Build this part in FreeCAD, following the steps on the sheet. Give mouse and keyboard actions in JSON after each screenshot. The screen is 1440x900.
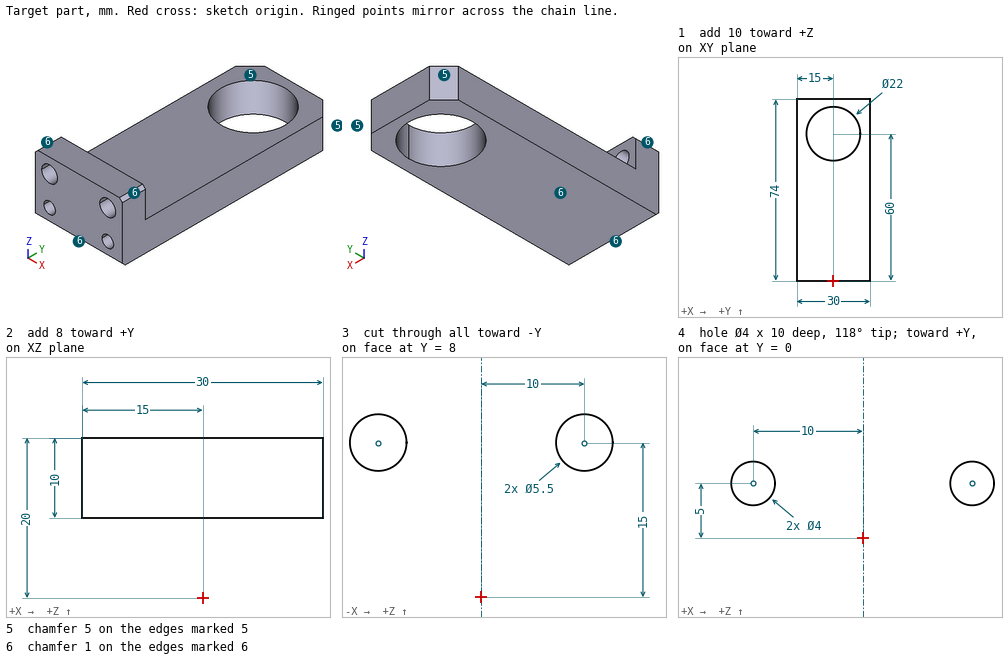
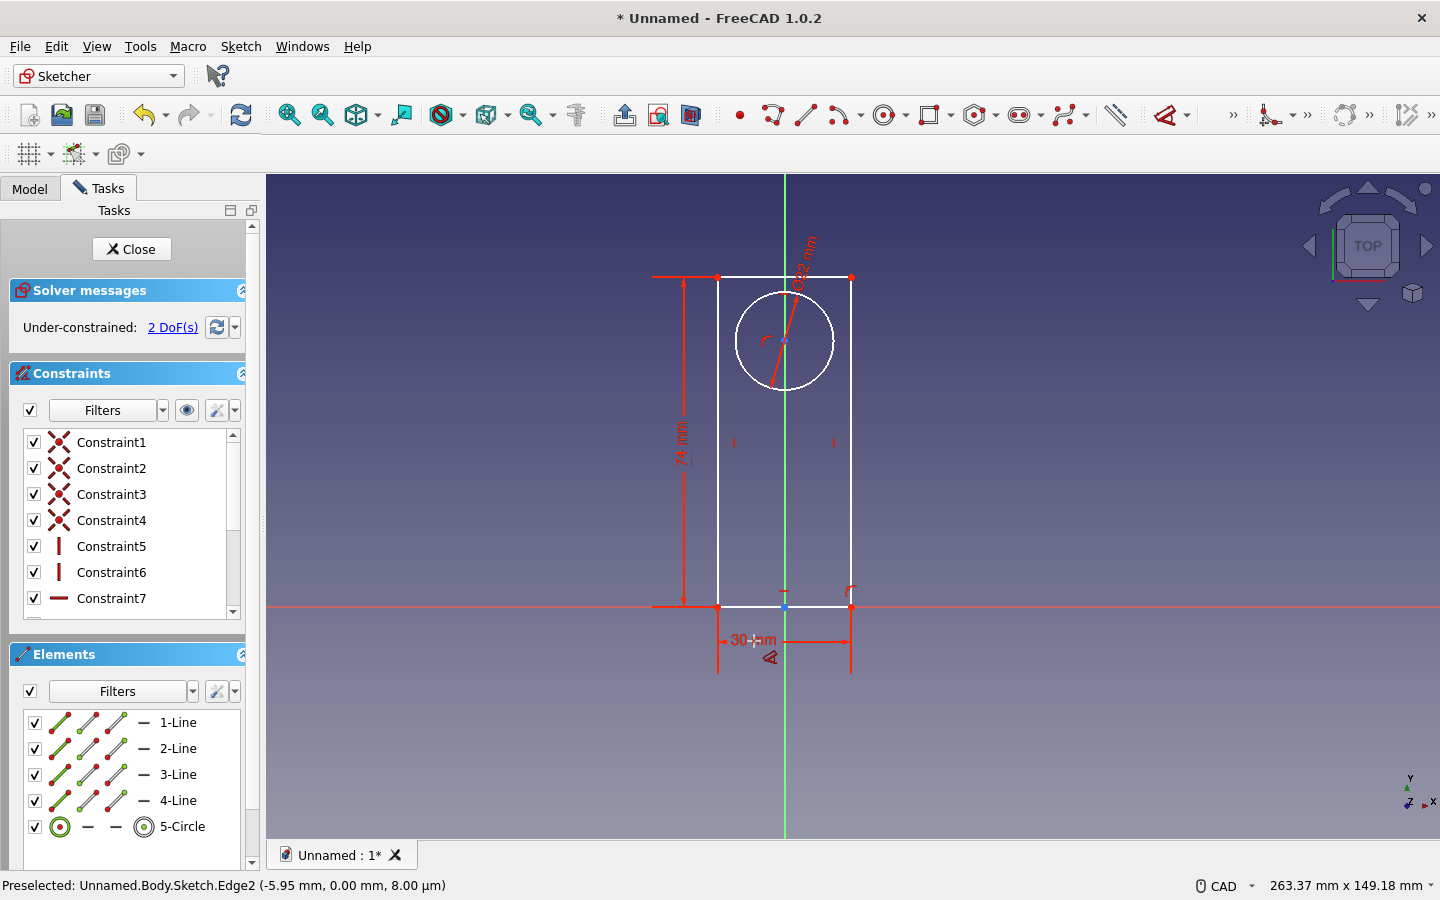
{"action": "left_click", "coordinate": [785, 341]}
{"action": "left_click", "coordinate": [819, 474]}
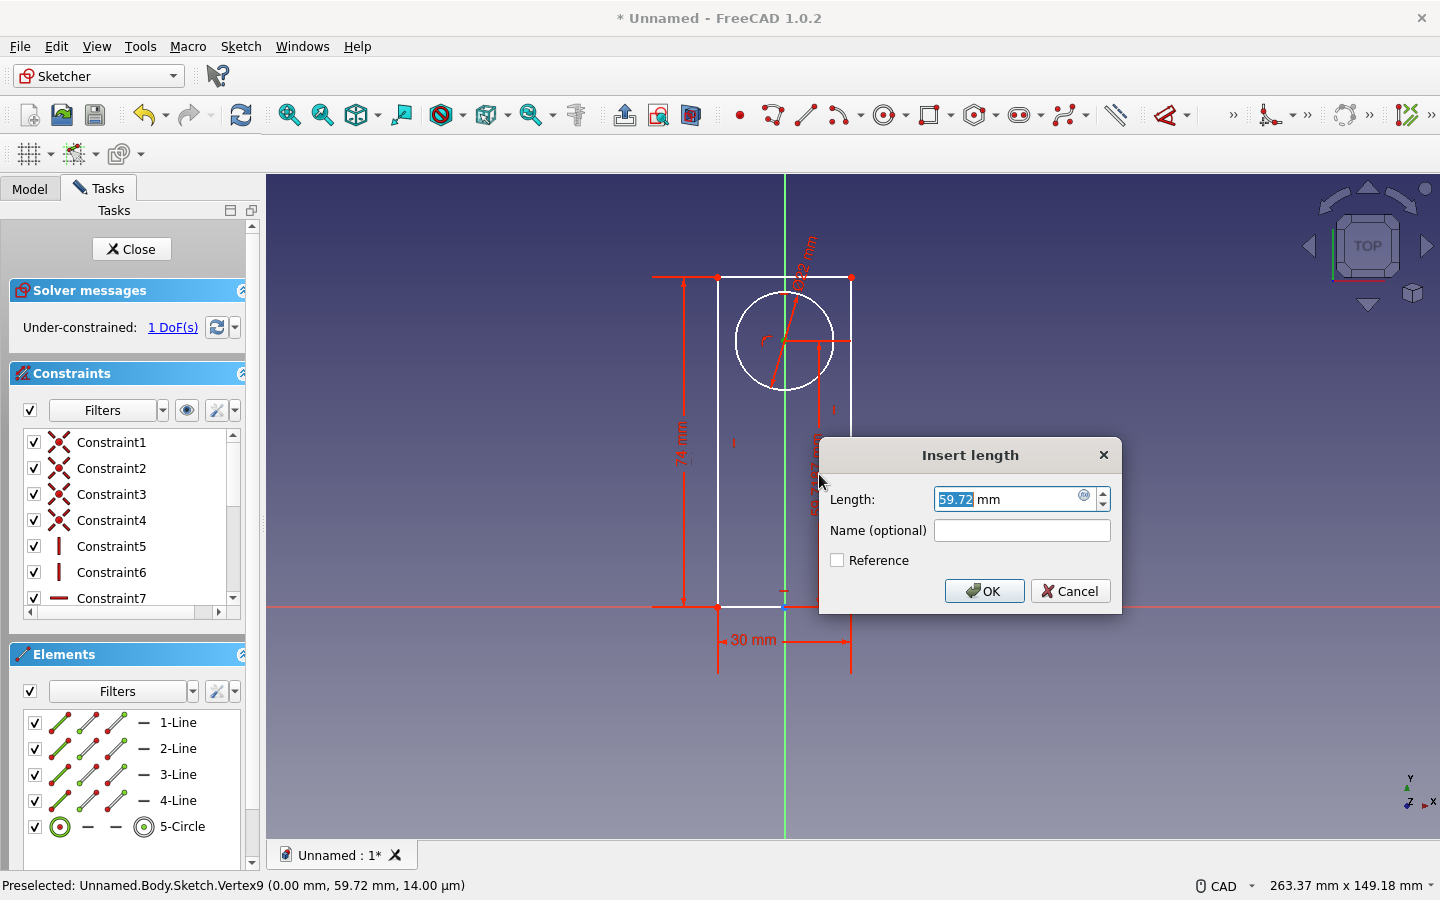
{"action": "type", "text": "60"}
{"action": "key", "text": "Return"}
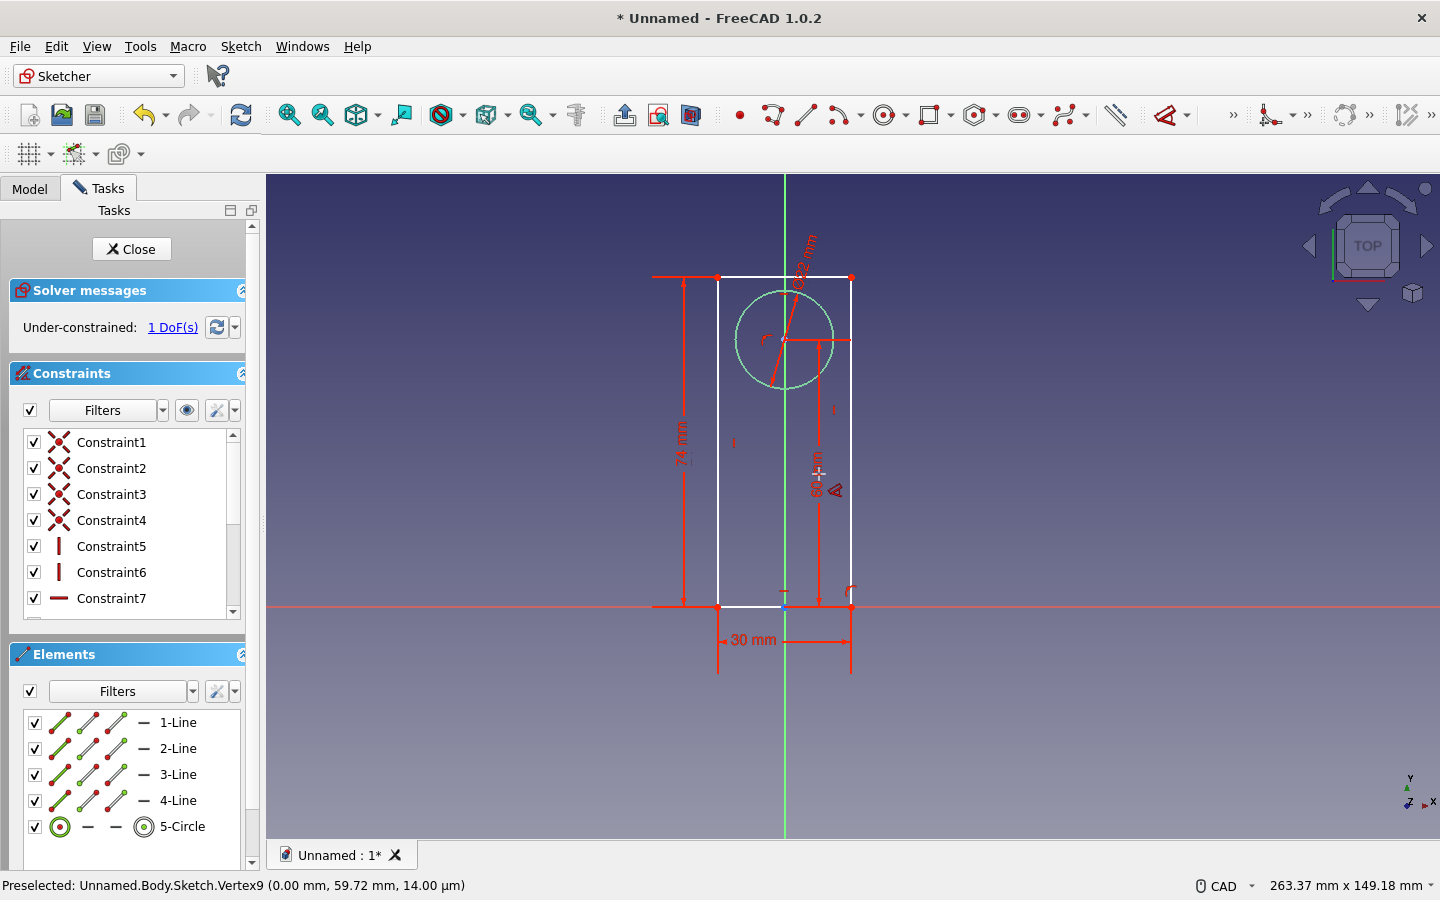
{"action": "left_click", "coordinate": [718, 277]}
{"action": "left_click", "coordinate": [736, 243]}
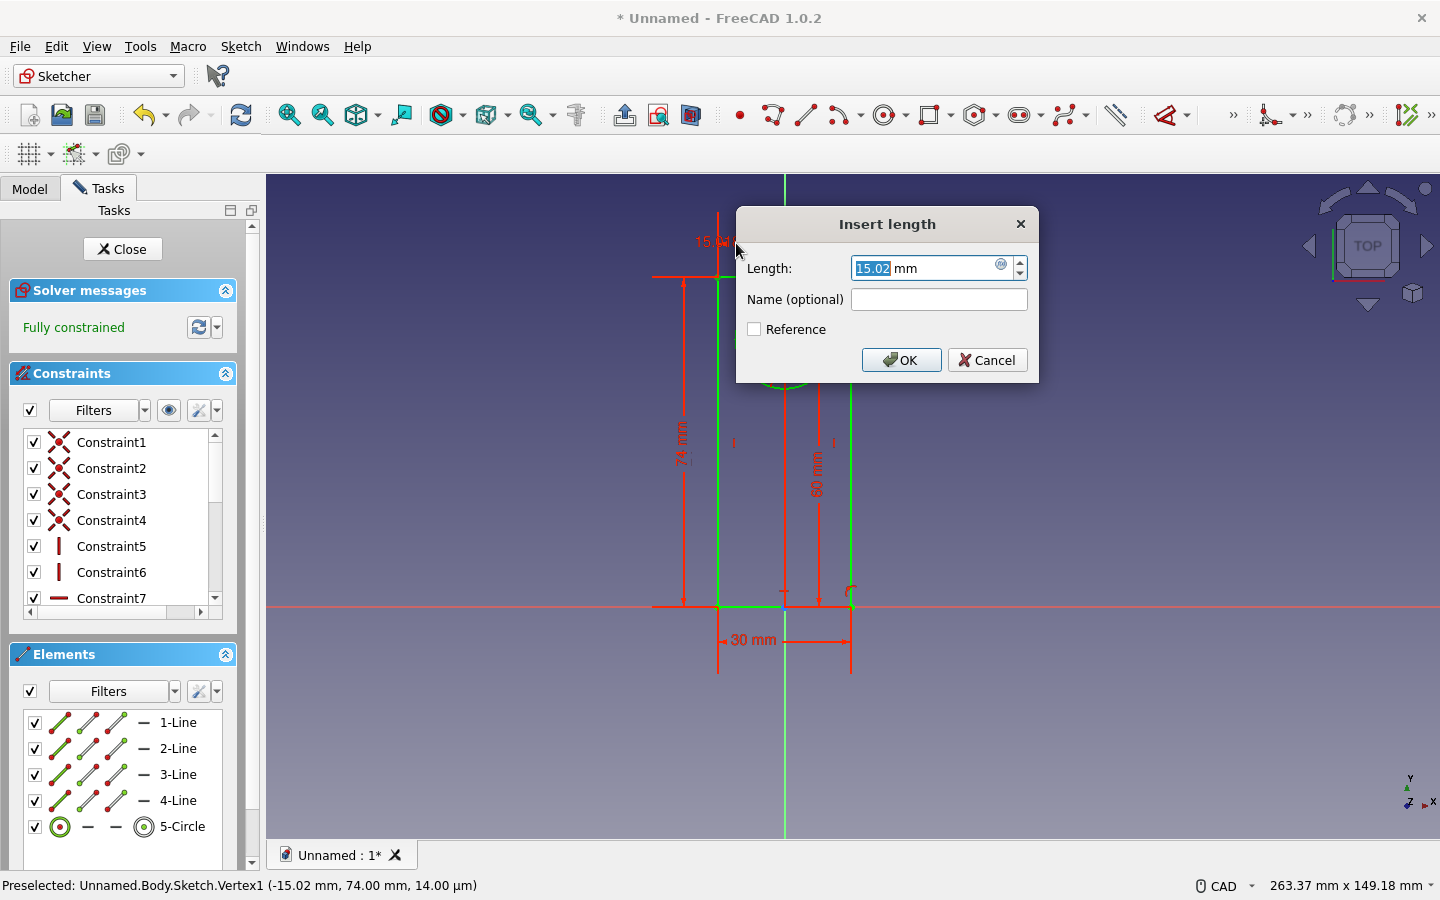
{"action": "type", "text": "15"}
{"action": "key", "text": "Return"}
{"action": "key", "text": "Escape"}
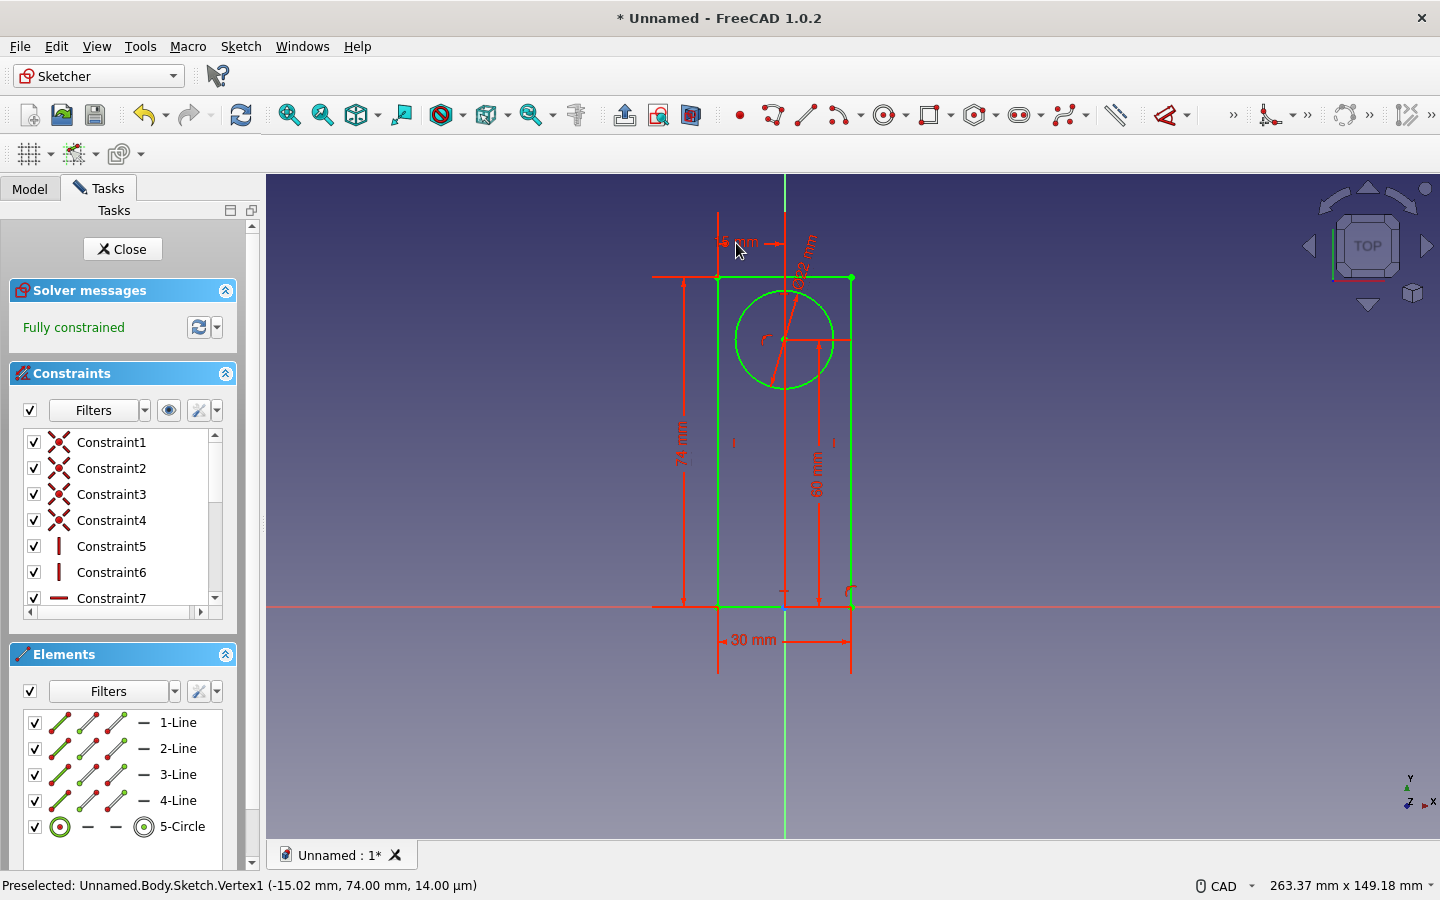
{"action": "left_click", "coordinate": [123, 249]}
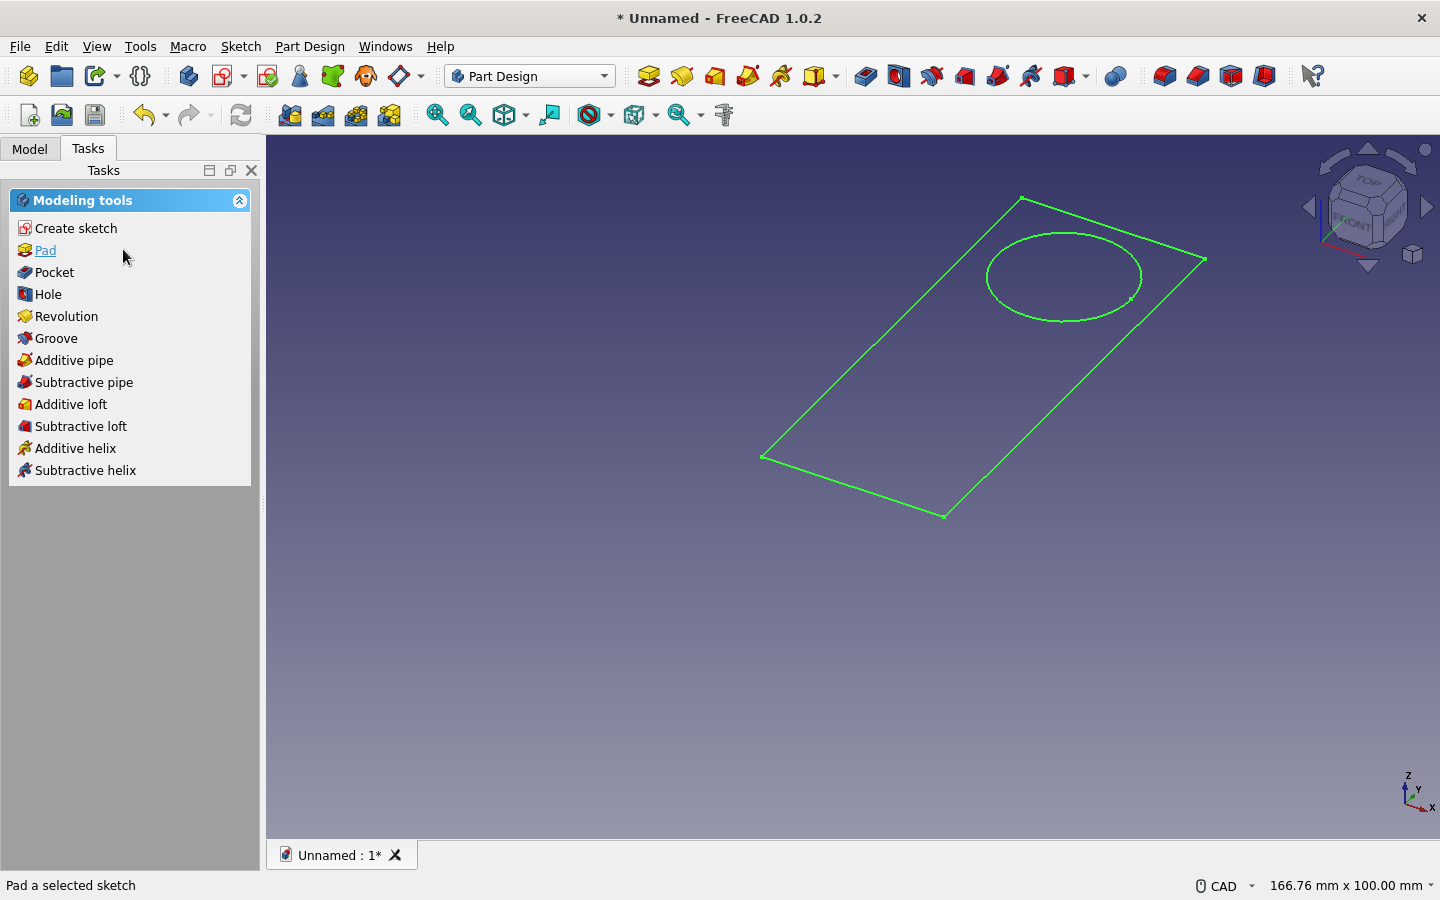
{"action": "left_click", "coordinate": [649, 76]}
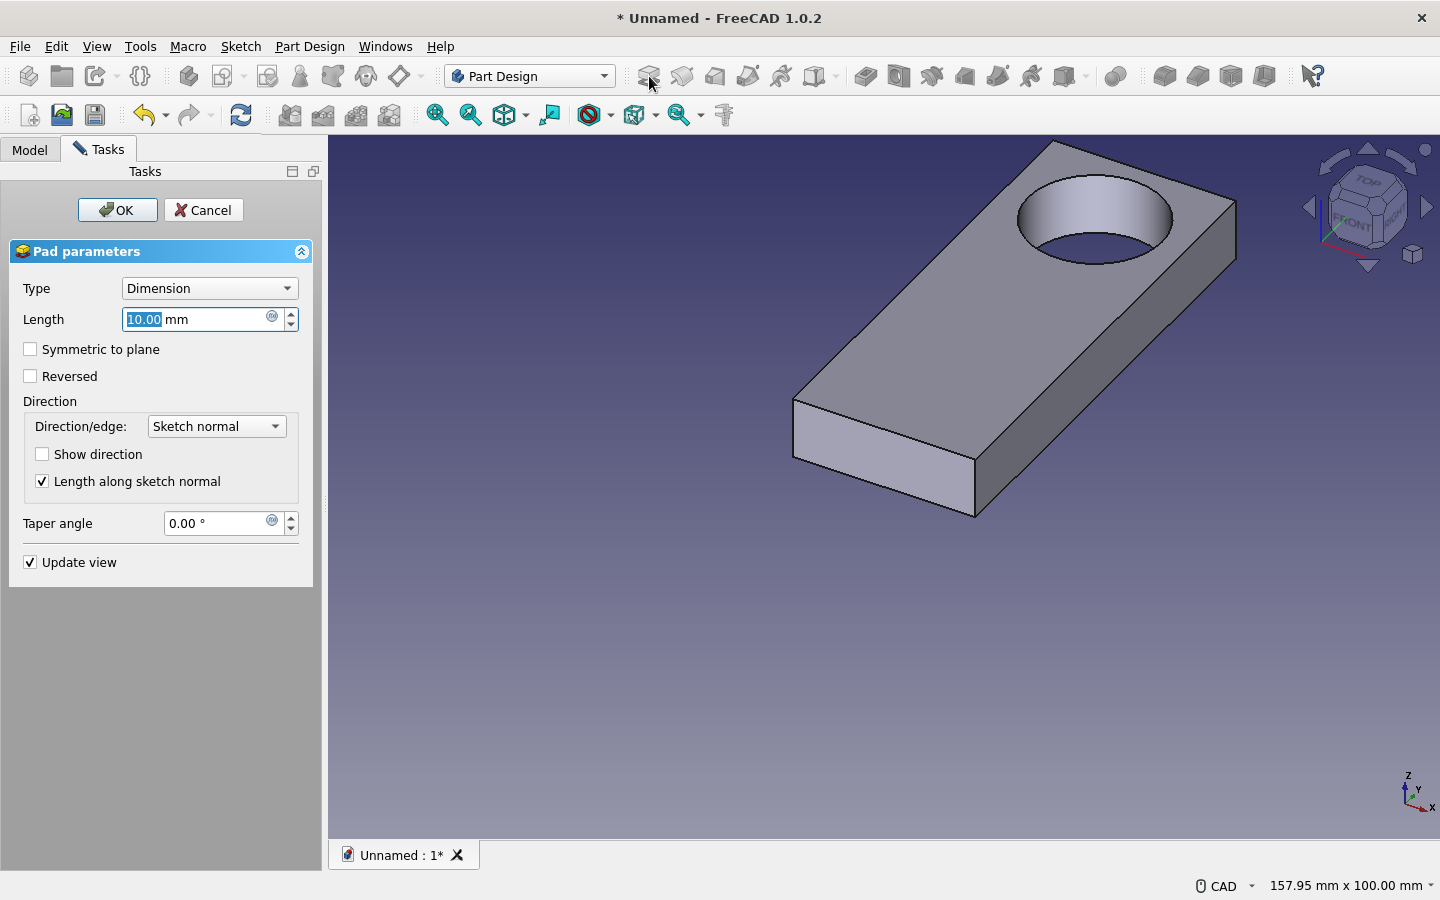
{"action": "type", "text": "10"}
{"action": "key", "text": "Tab"}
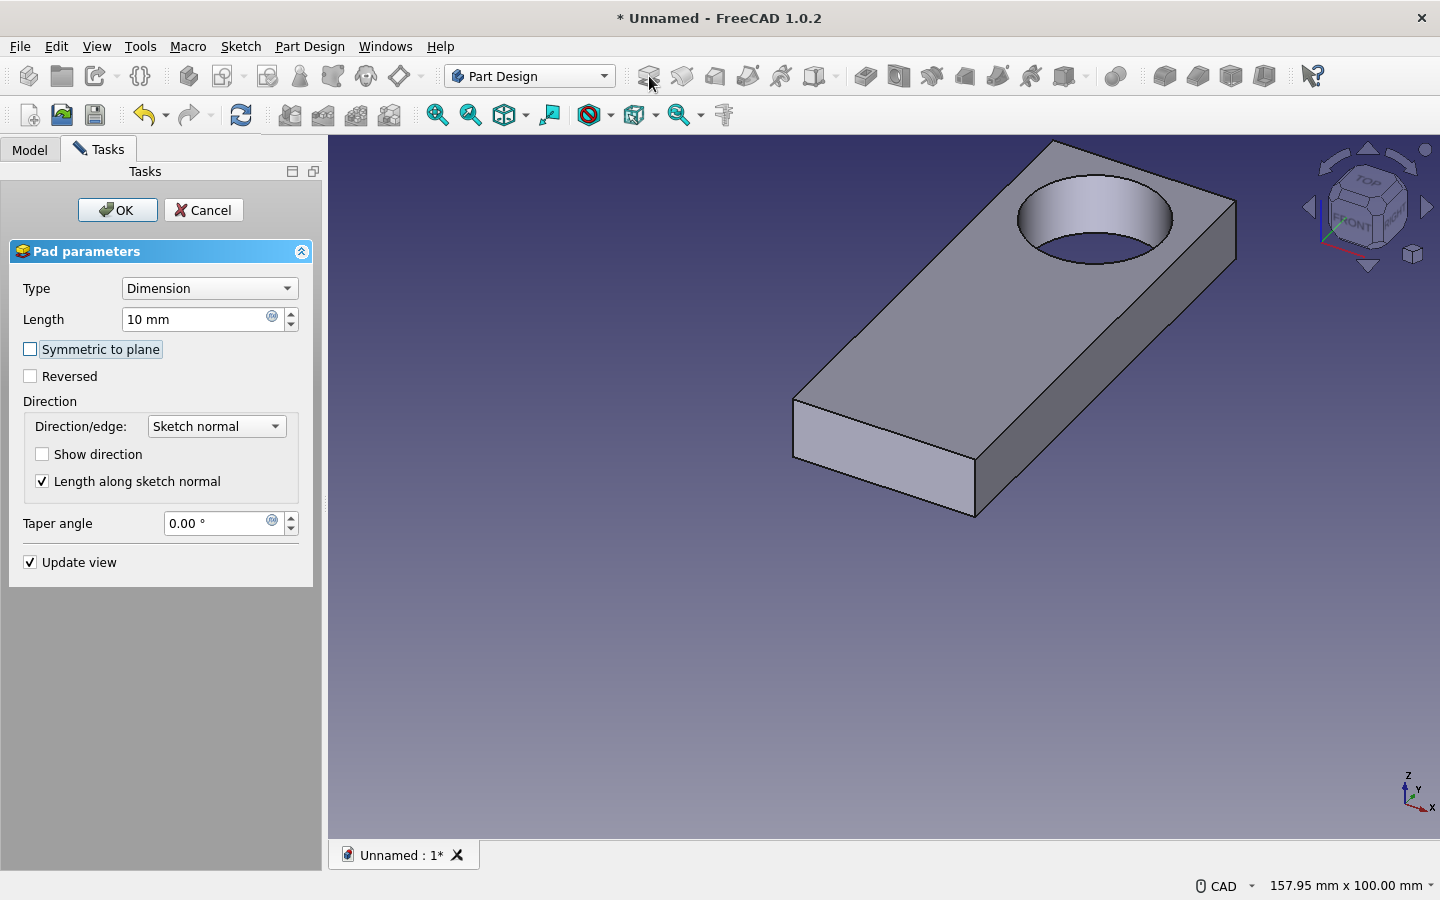
{"action": "left_click", "coordinate": [118, 210]}